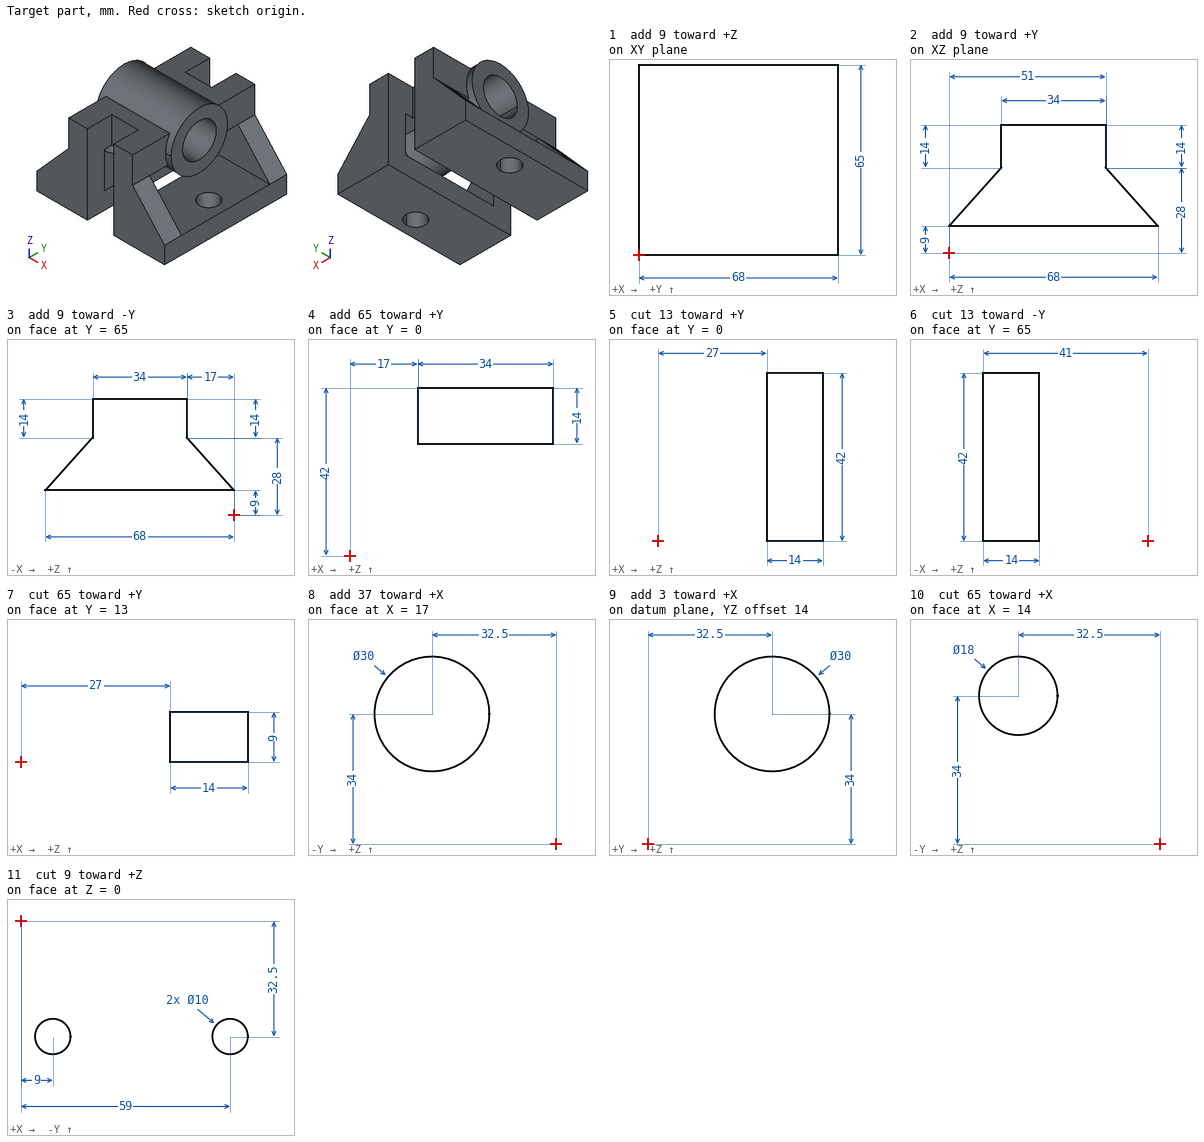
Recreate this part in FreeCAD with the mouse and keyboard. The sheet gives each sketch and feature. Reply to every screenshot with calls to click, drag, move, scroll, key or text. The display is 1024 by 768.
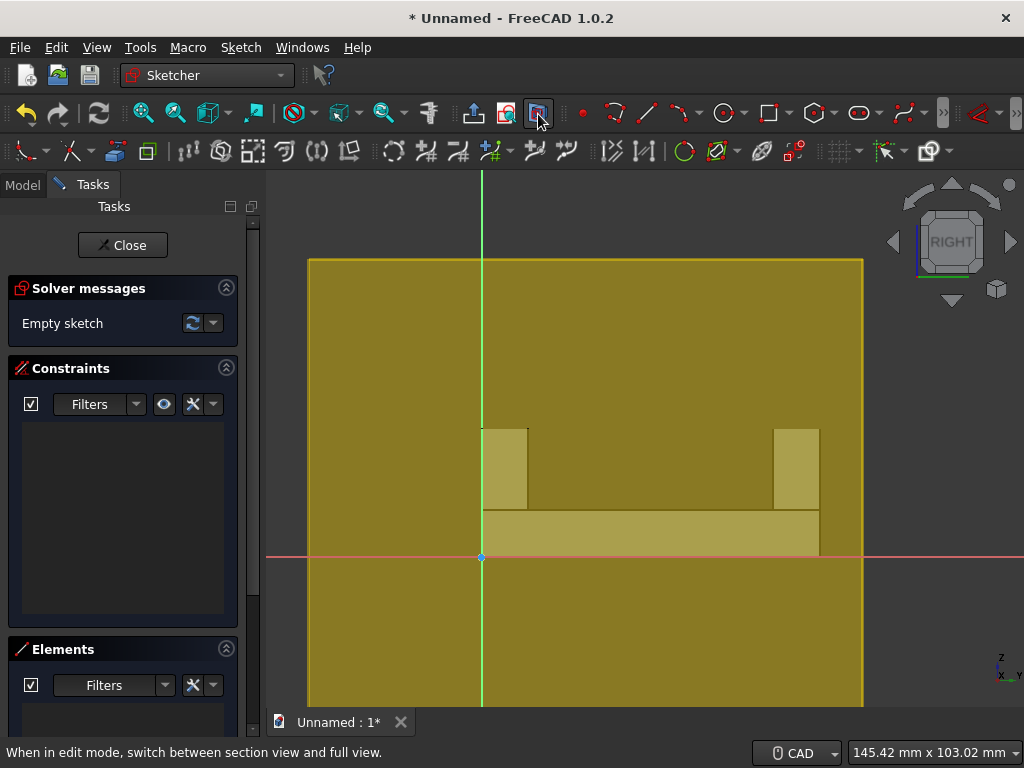
click(724, 114)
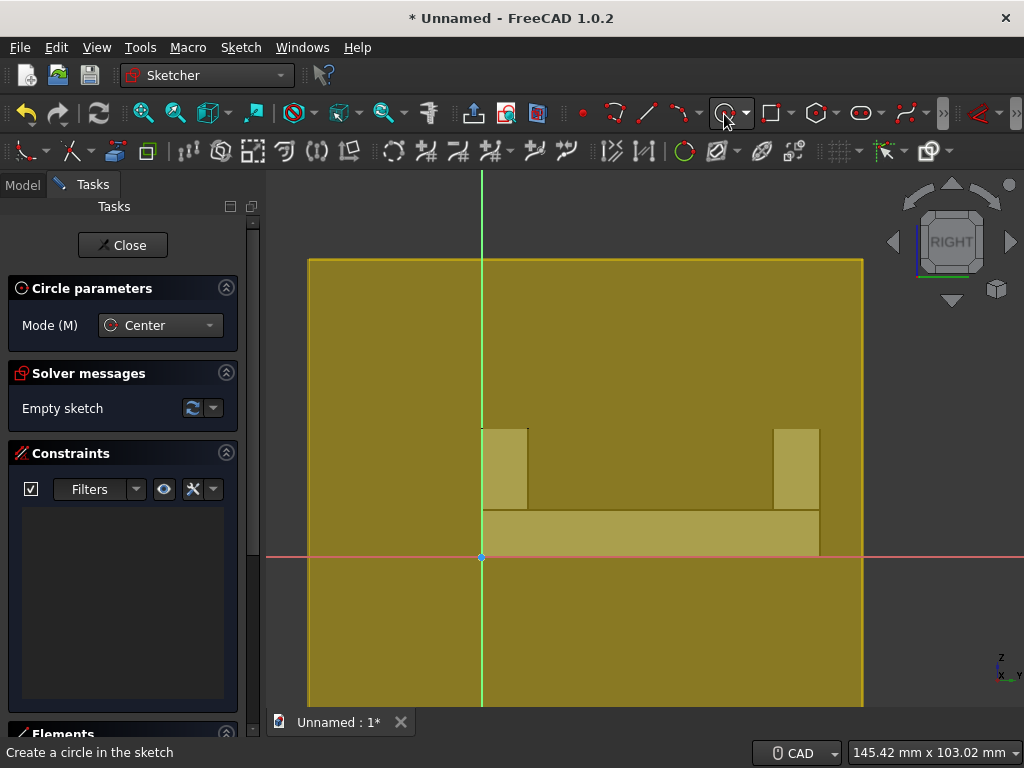
click(651, 380)
move(706, 325)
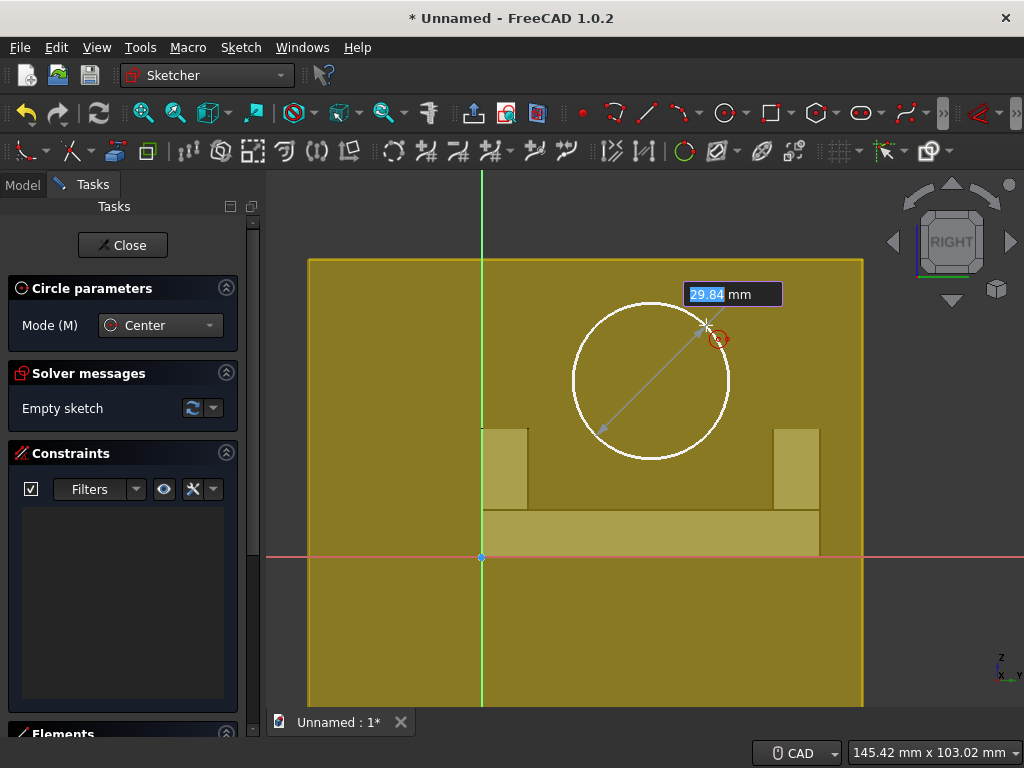
text(30)
key(Return)
key(Escape)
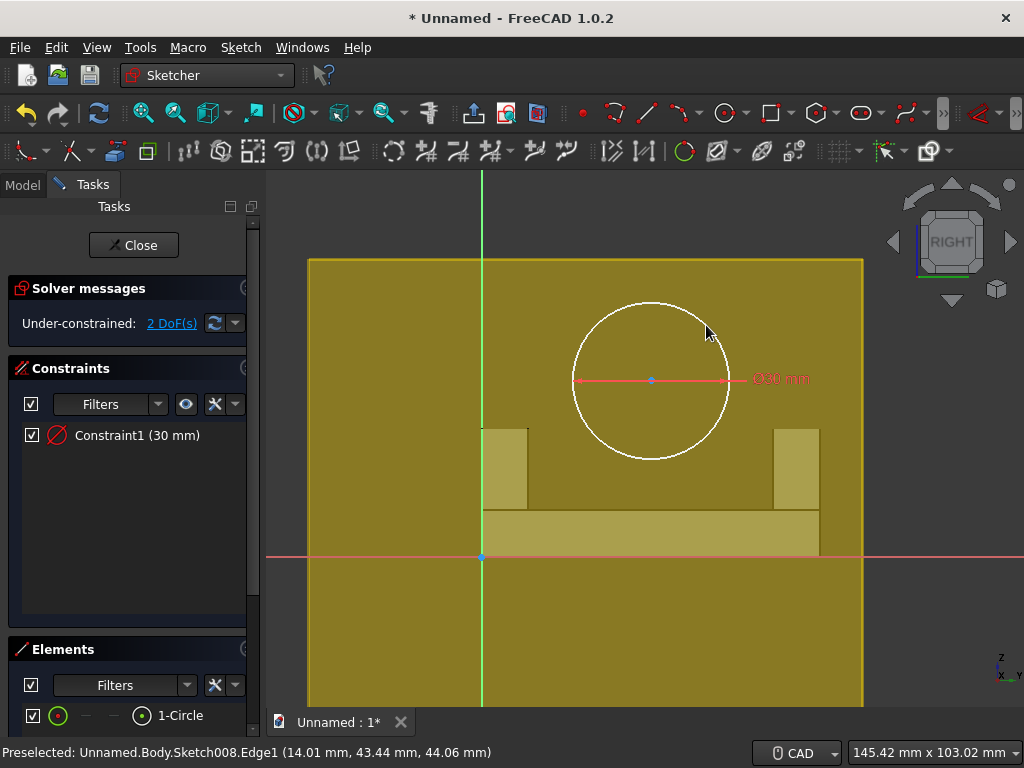
key(d)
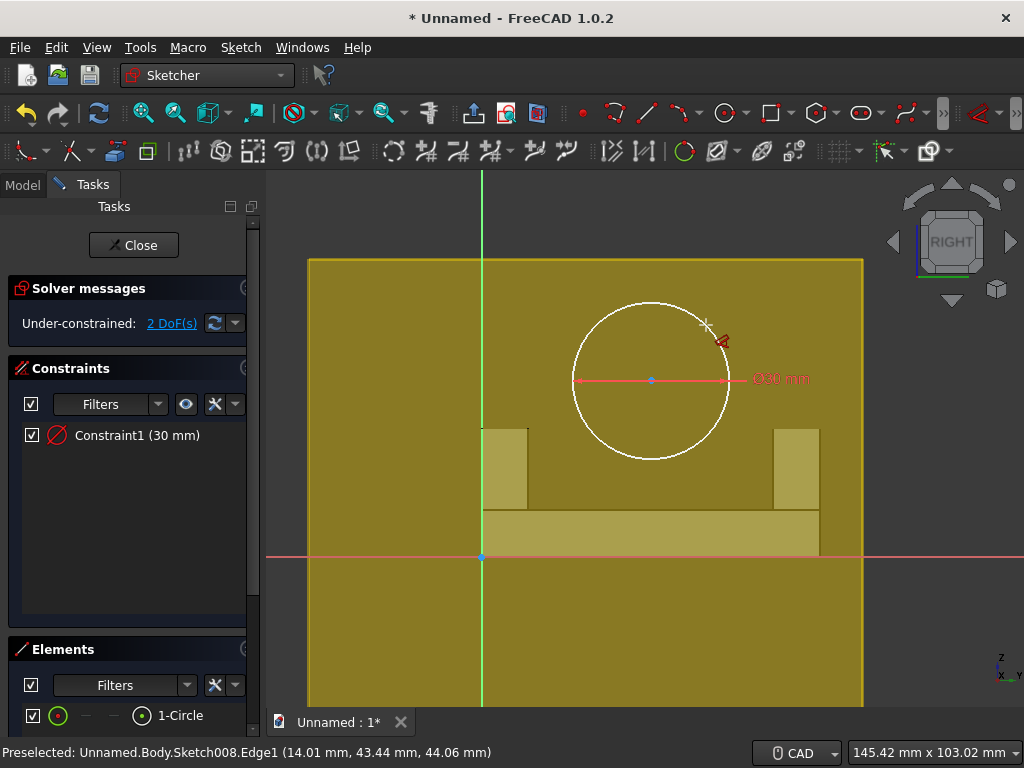
click(651, 381)
click(448, 469)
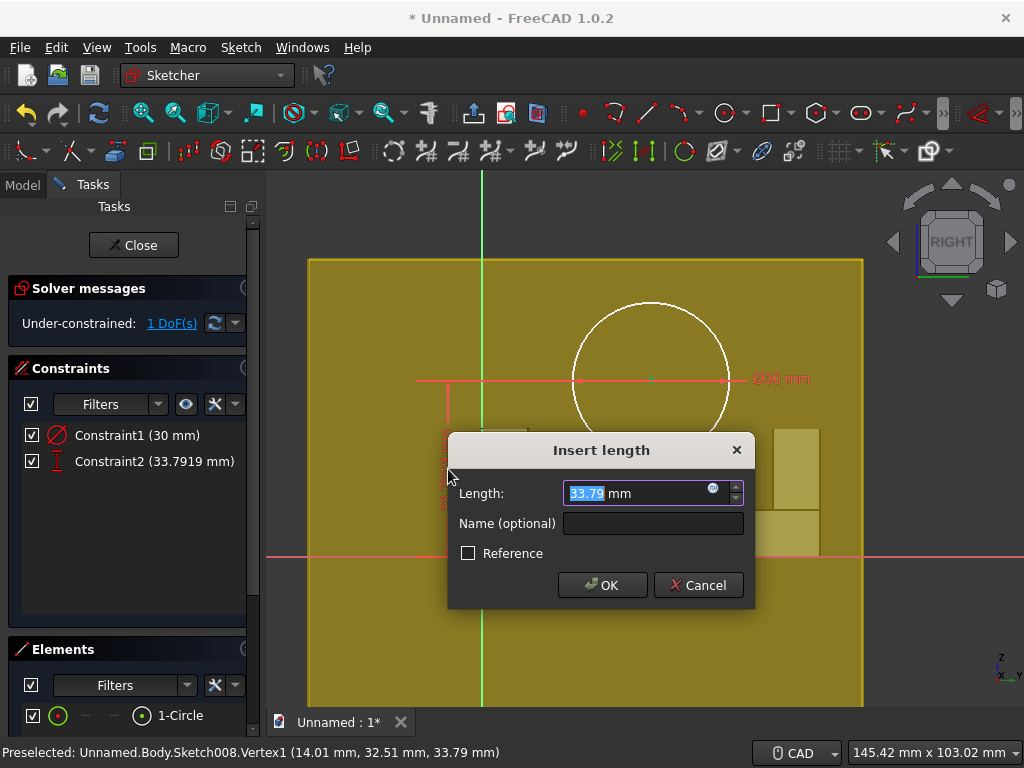
text(34)
key(Return)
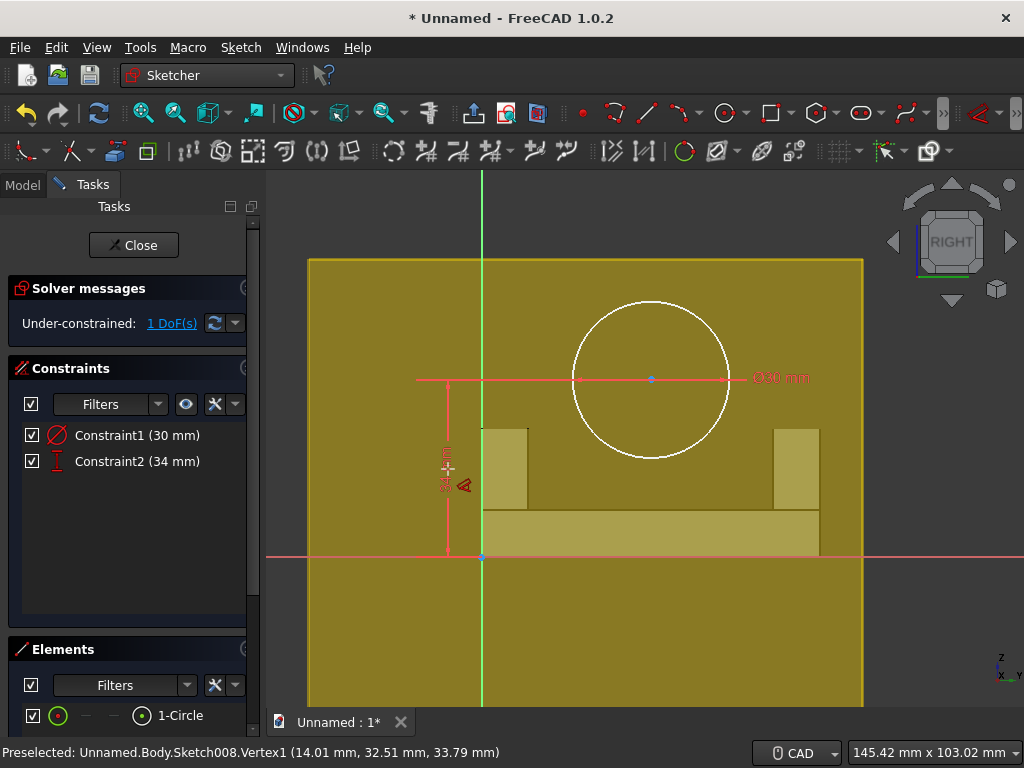
click(651, 380)
click(566, 591)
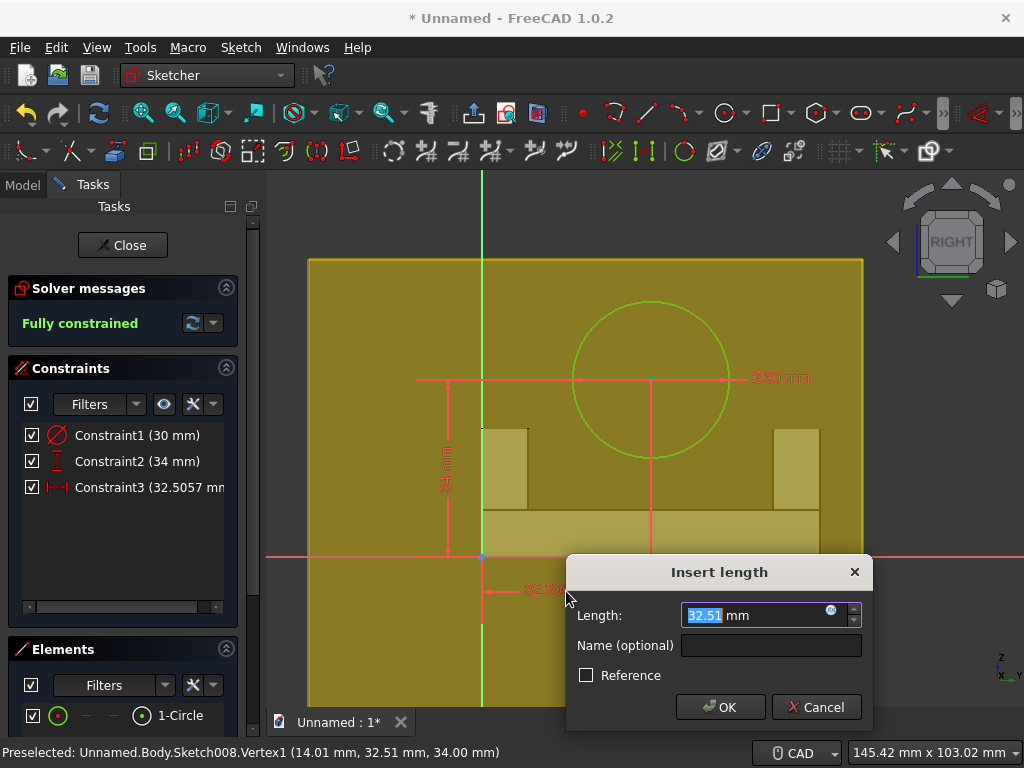
text(32.5)
key(Return)
key(Escape)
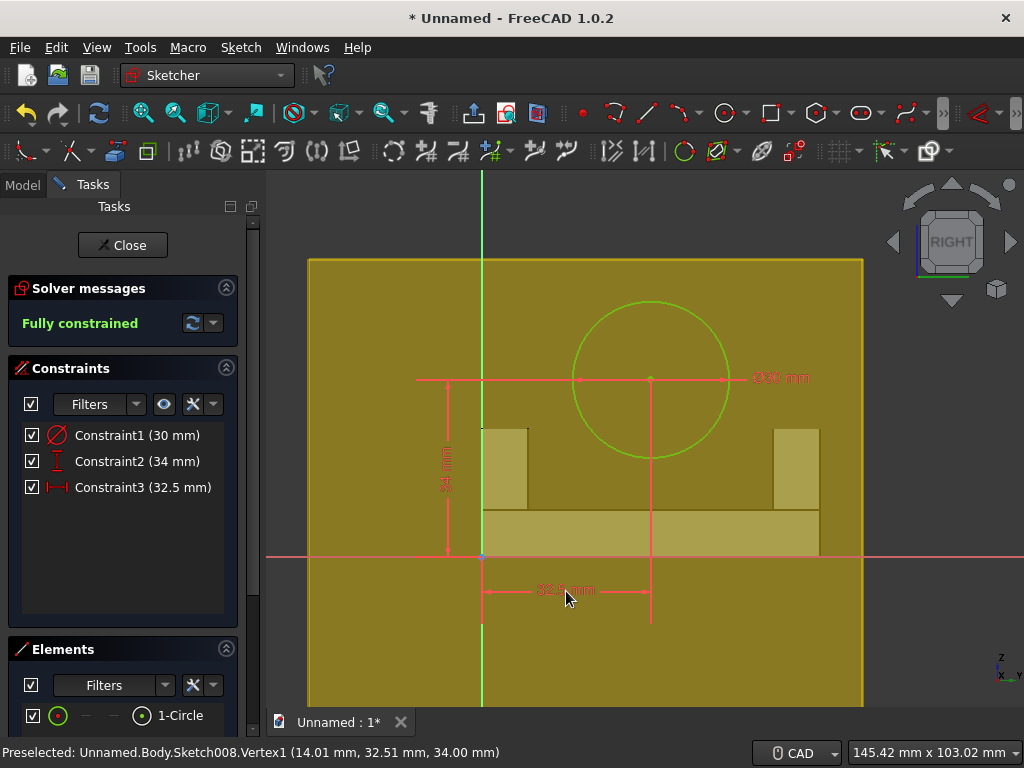
click(123, 245)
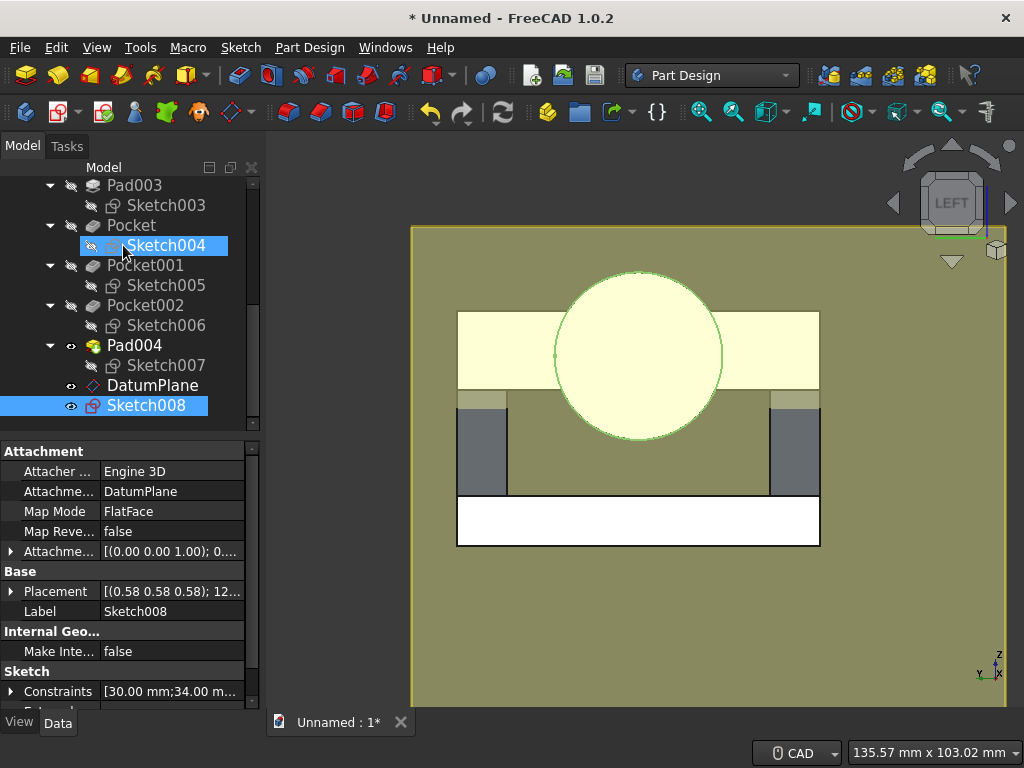
click(26, 76)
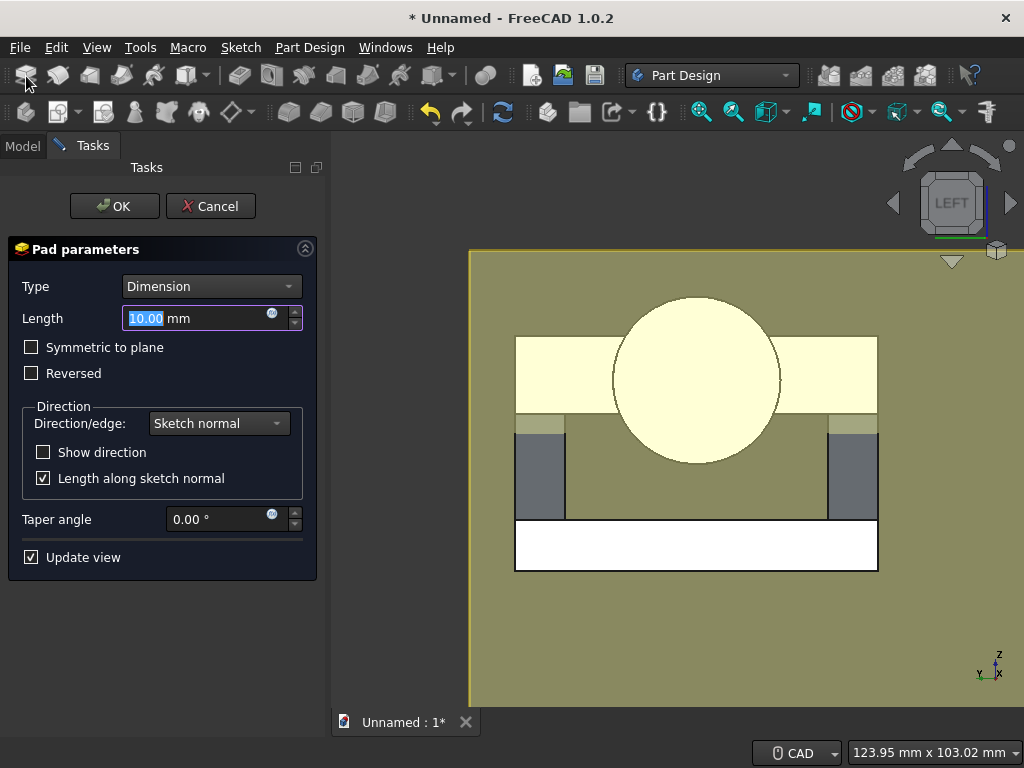
text(3)
key(Tab)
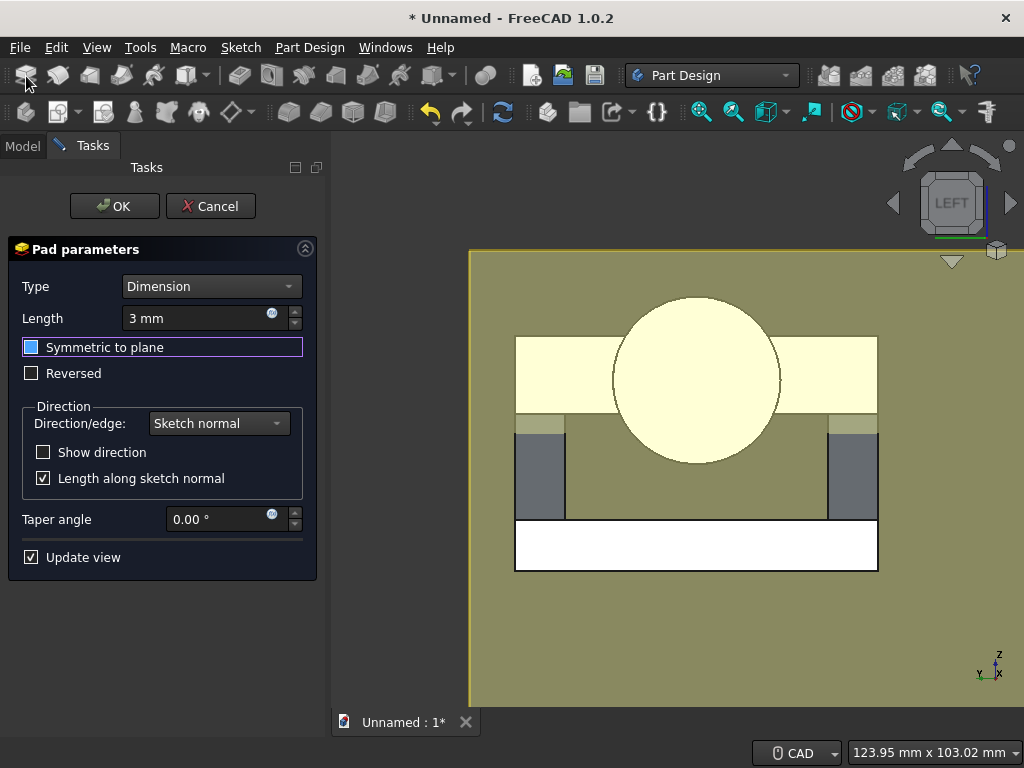
click(115, 206)